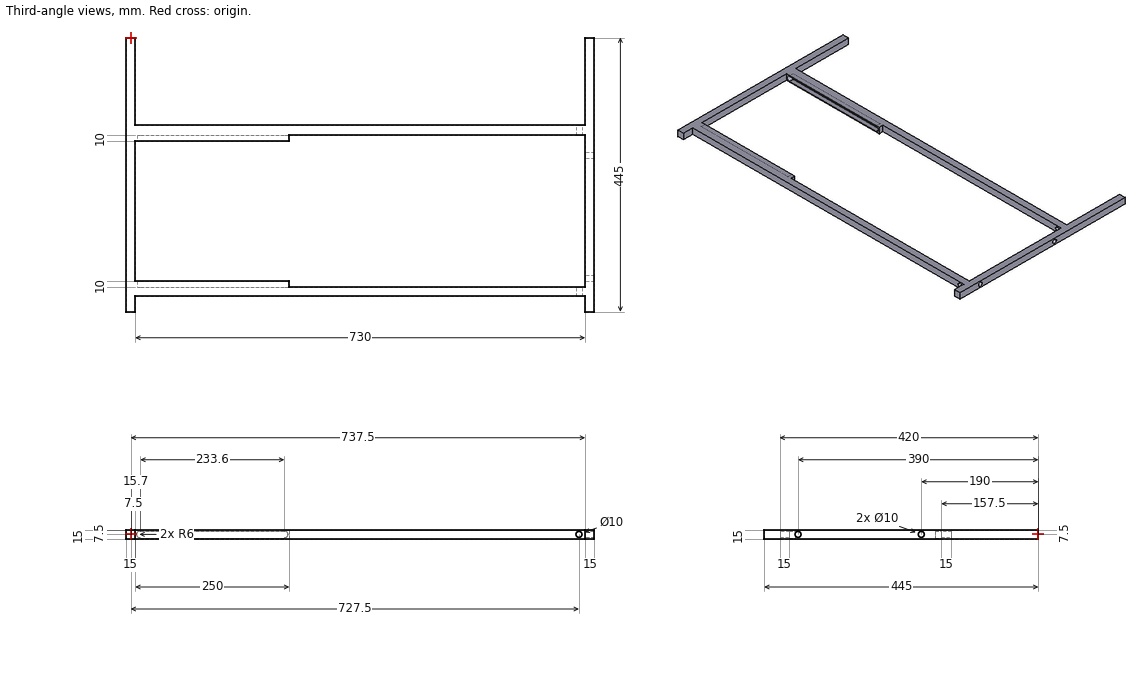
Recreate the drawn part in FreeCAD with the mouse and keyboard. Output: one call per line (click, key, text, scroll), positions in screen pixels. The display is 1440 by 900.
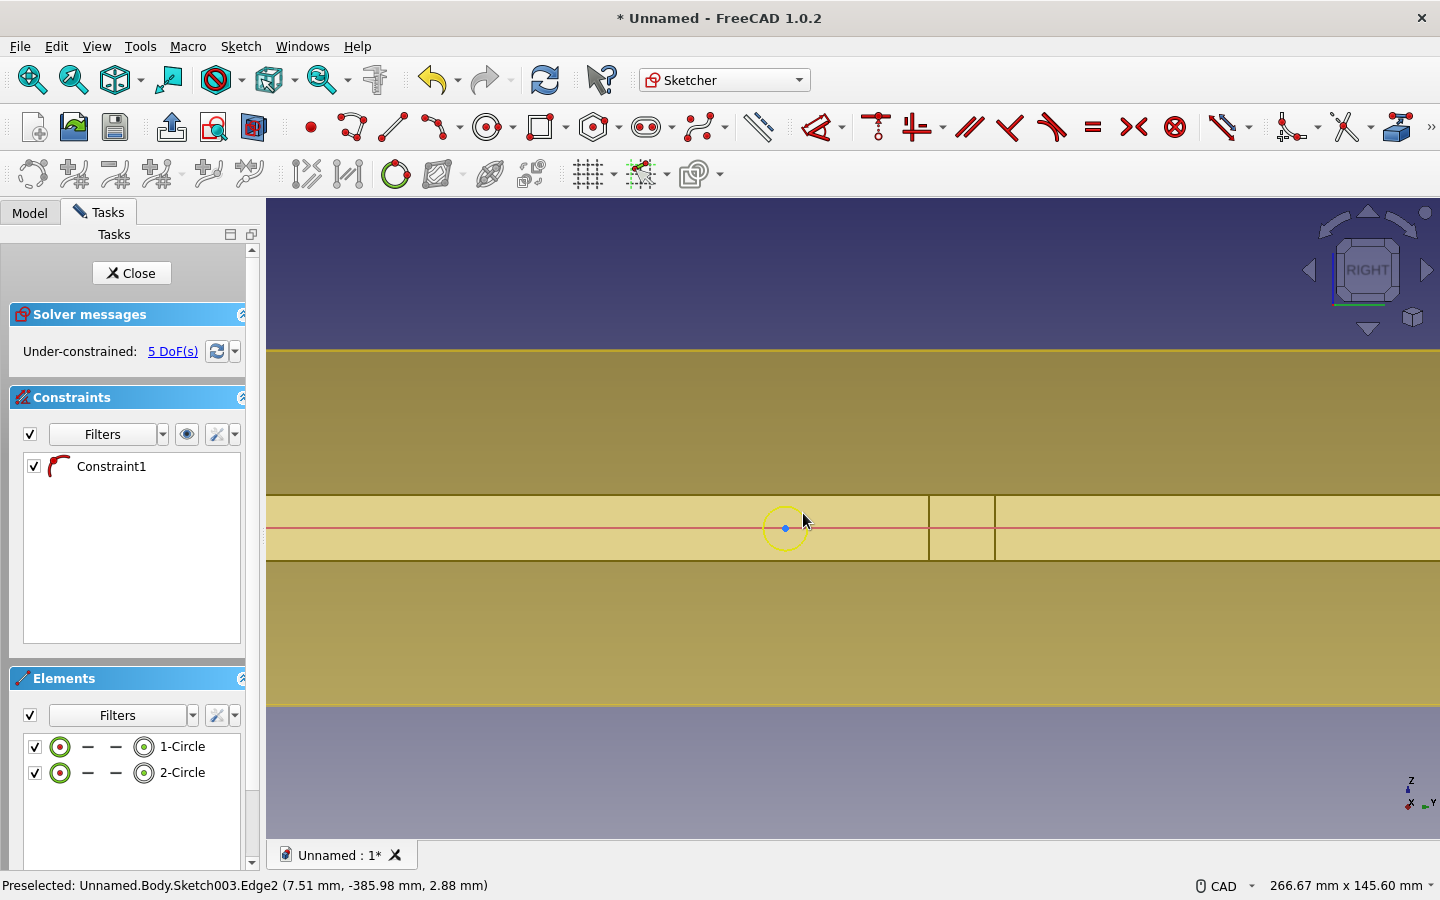
click(801, 513)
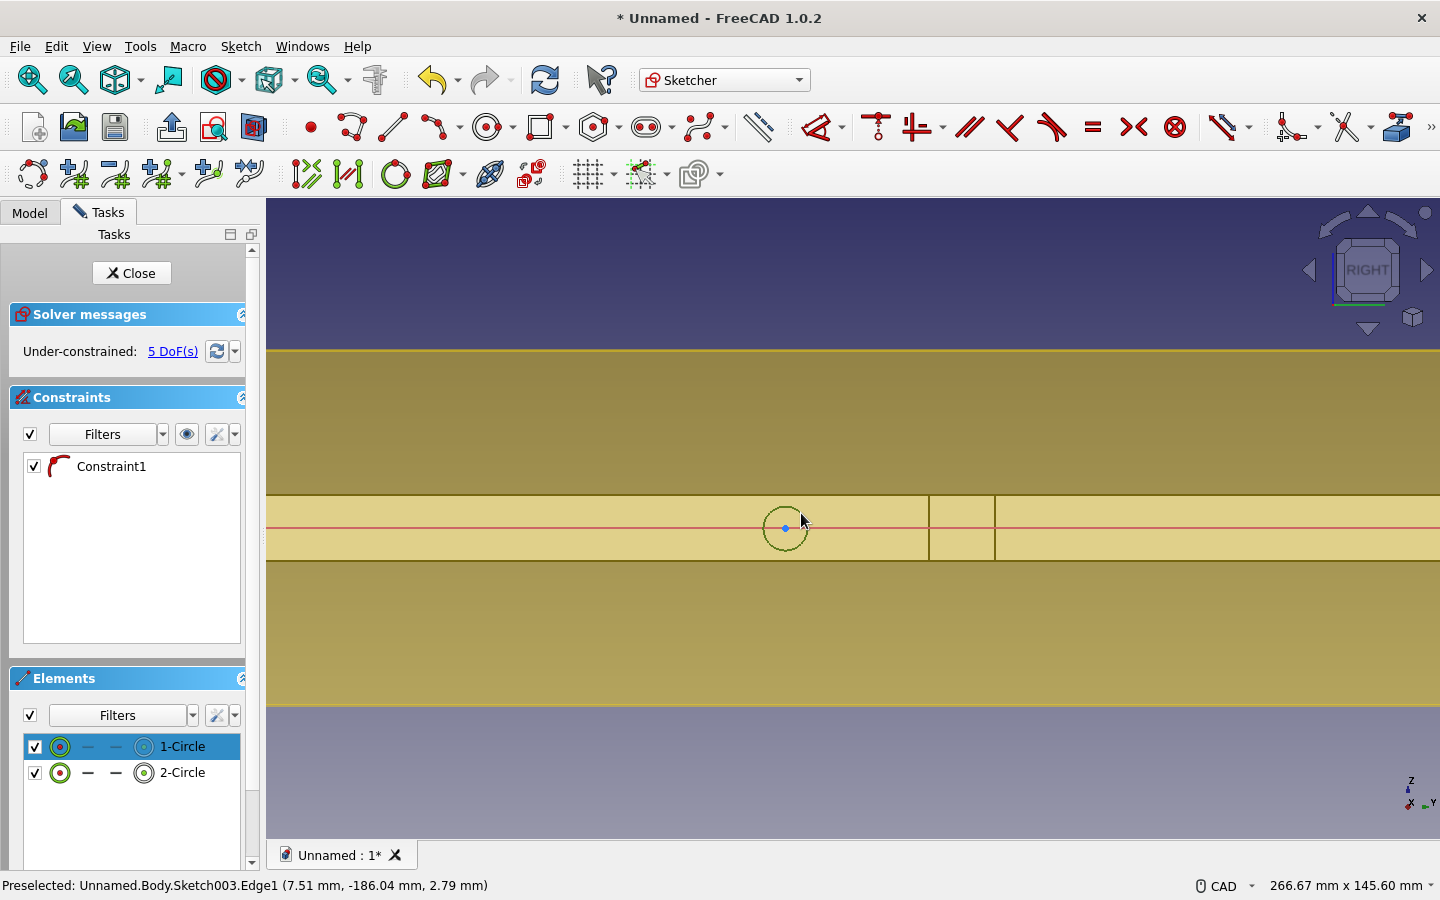
scroll(803, 513, down, 5)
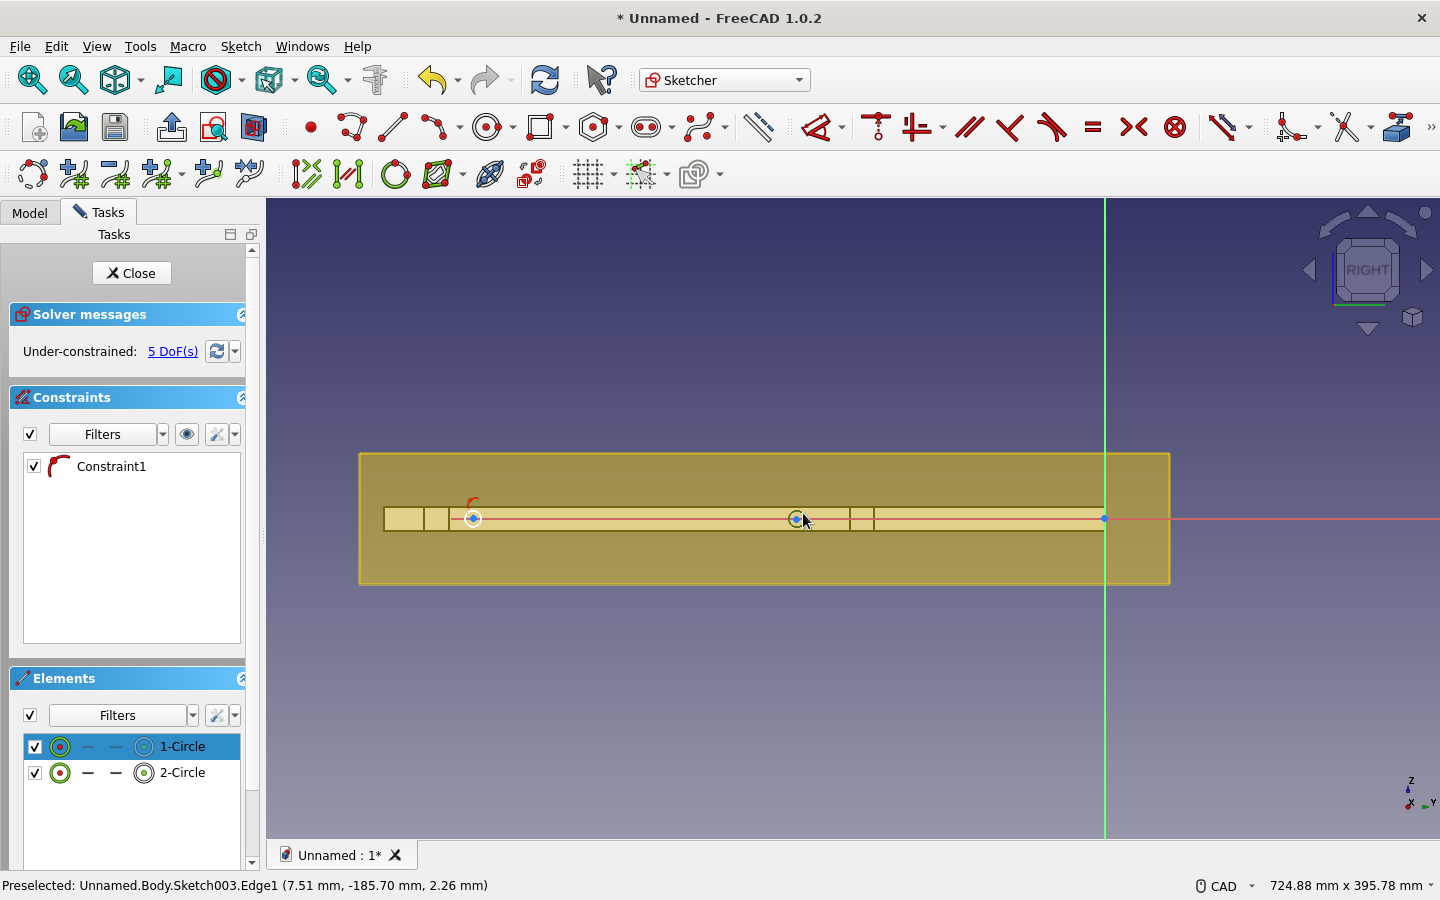
scroll(479, 513, up, 5)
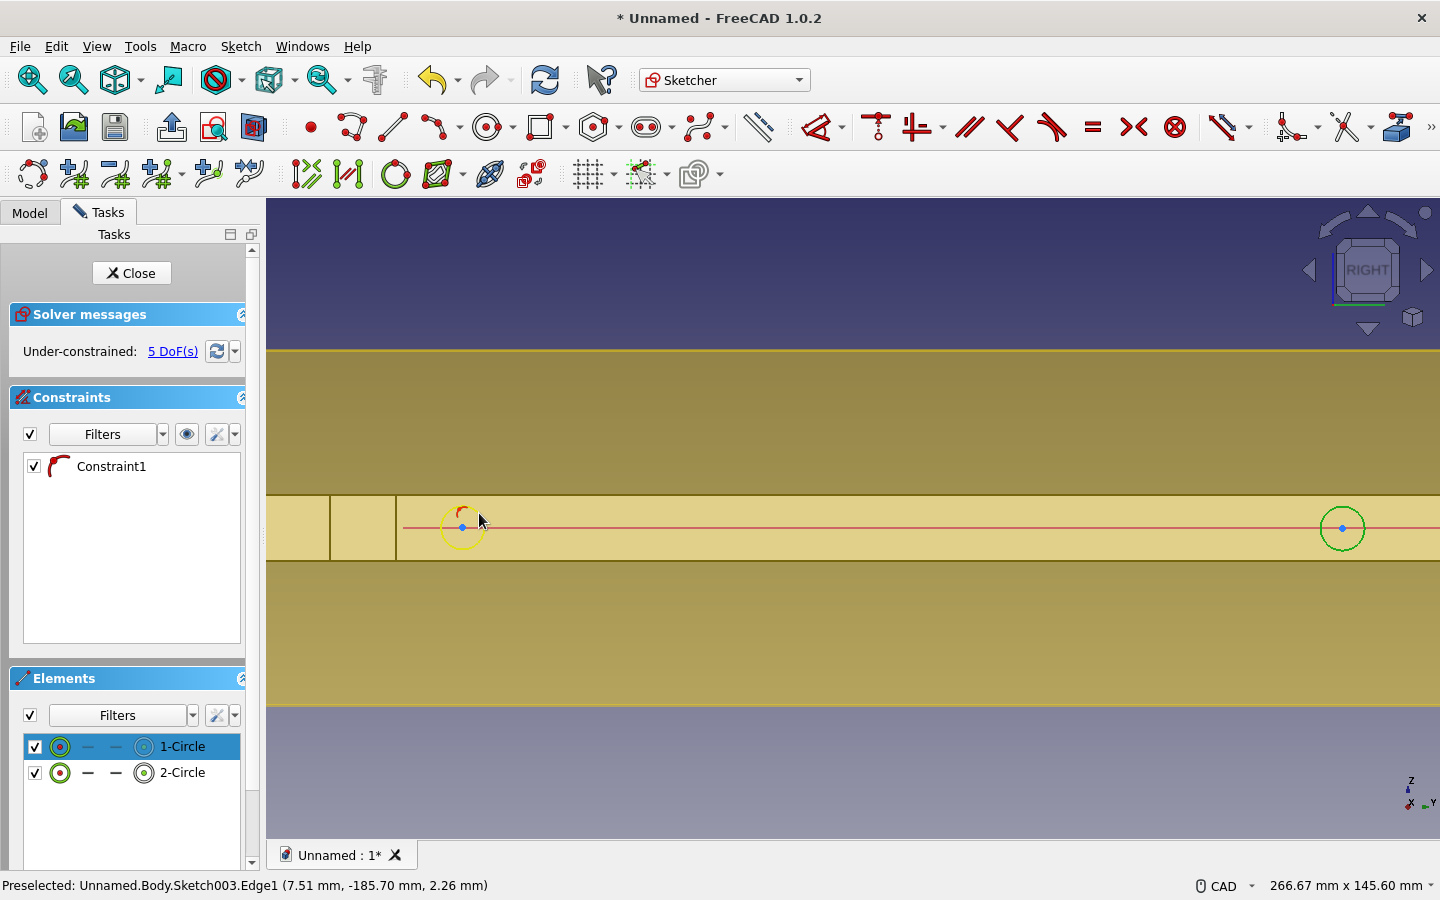
click(478, 513)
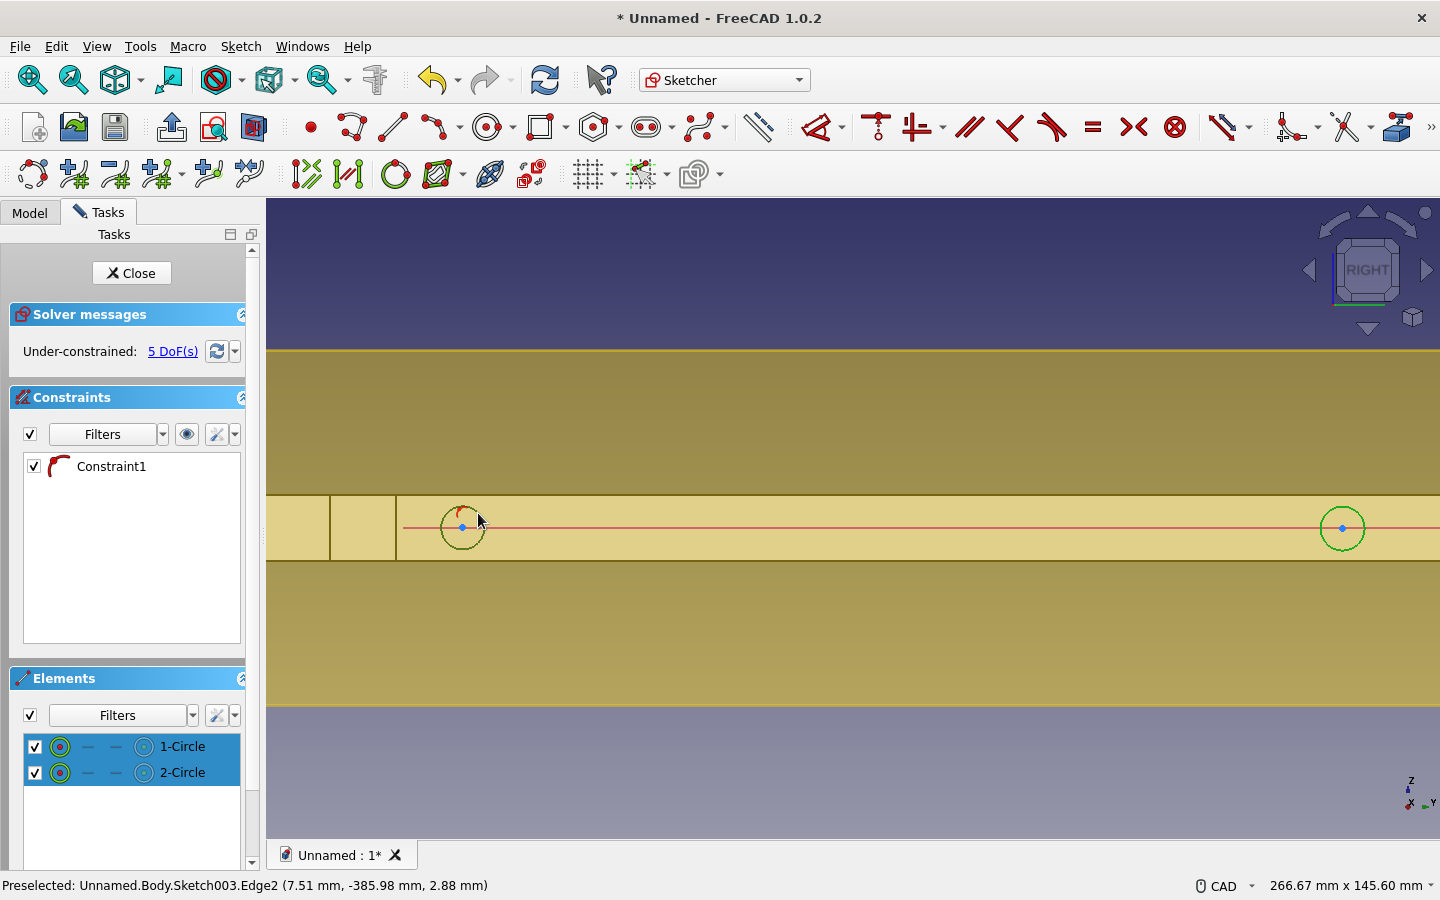
click(1093, 128)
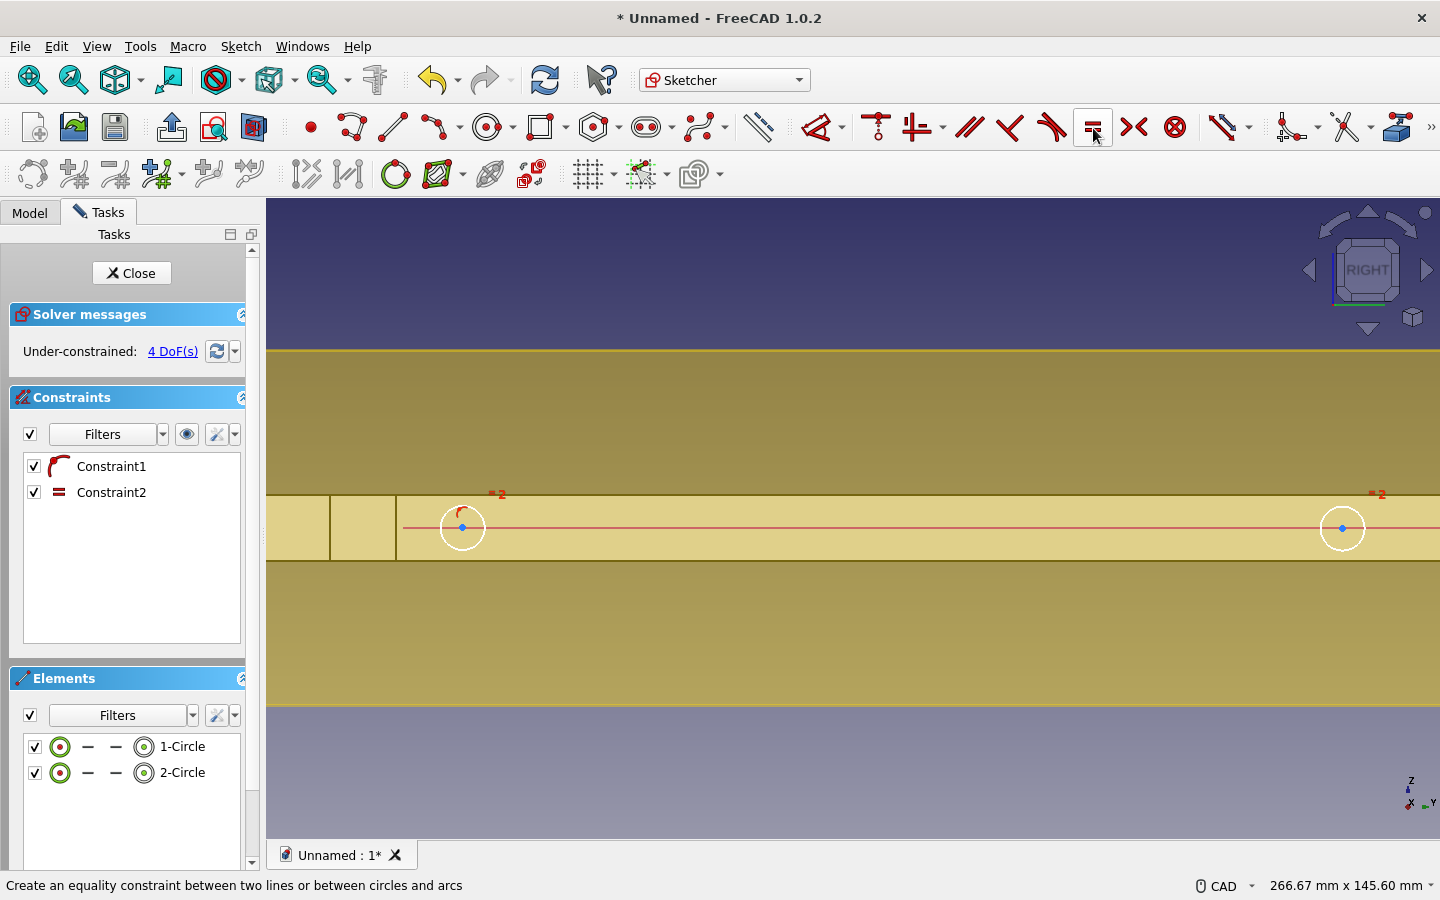
scroll(479, 513, down, 5)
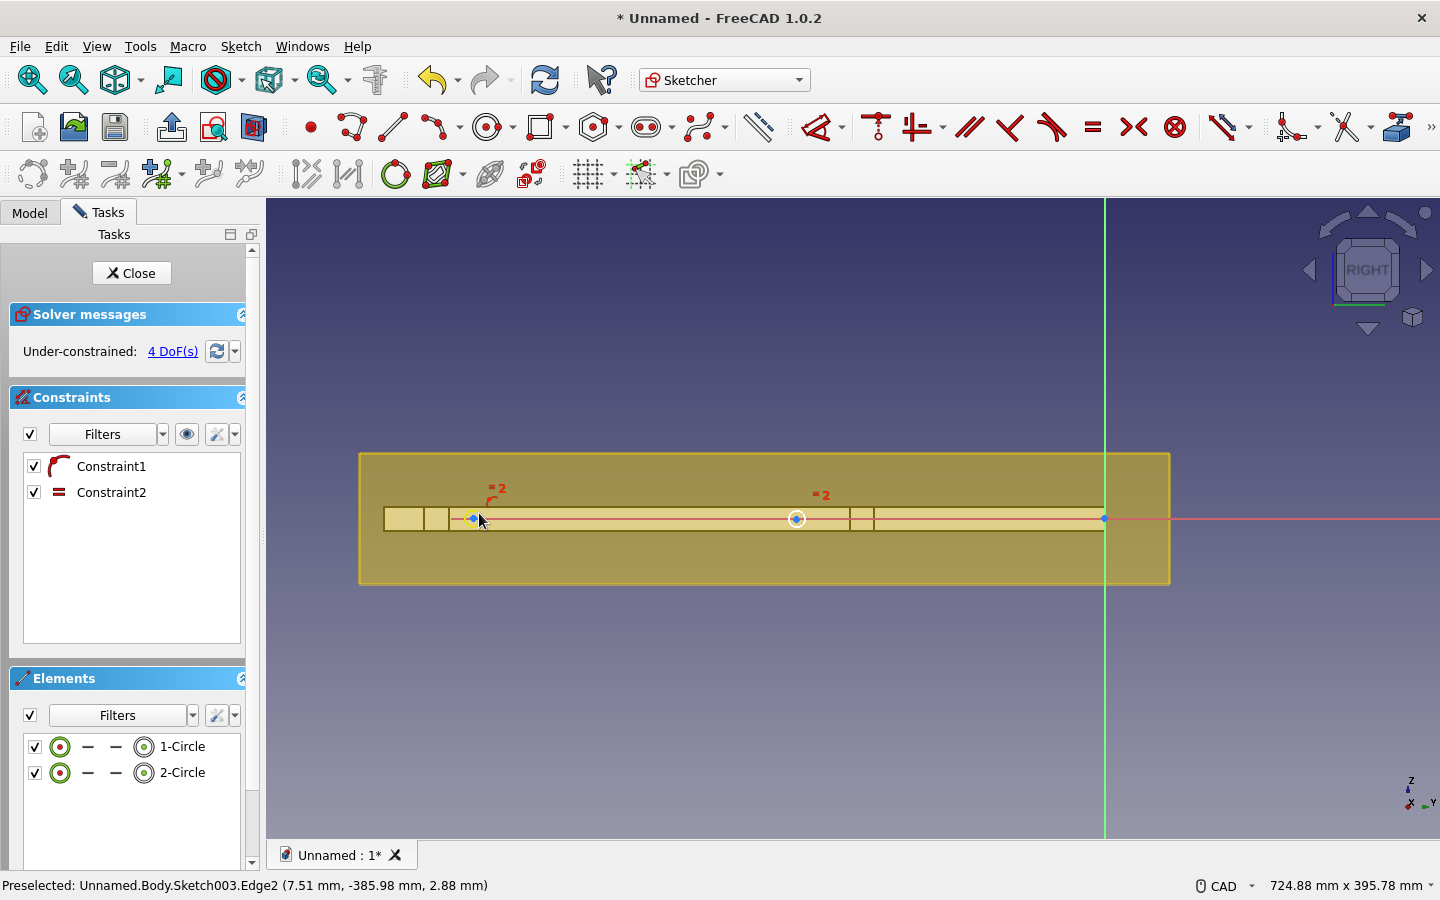
click(797, 519)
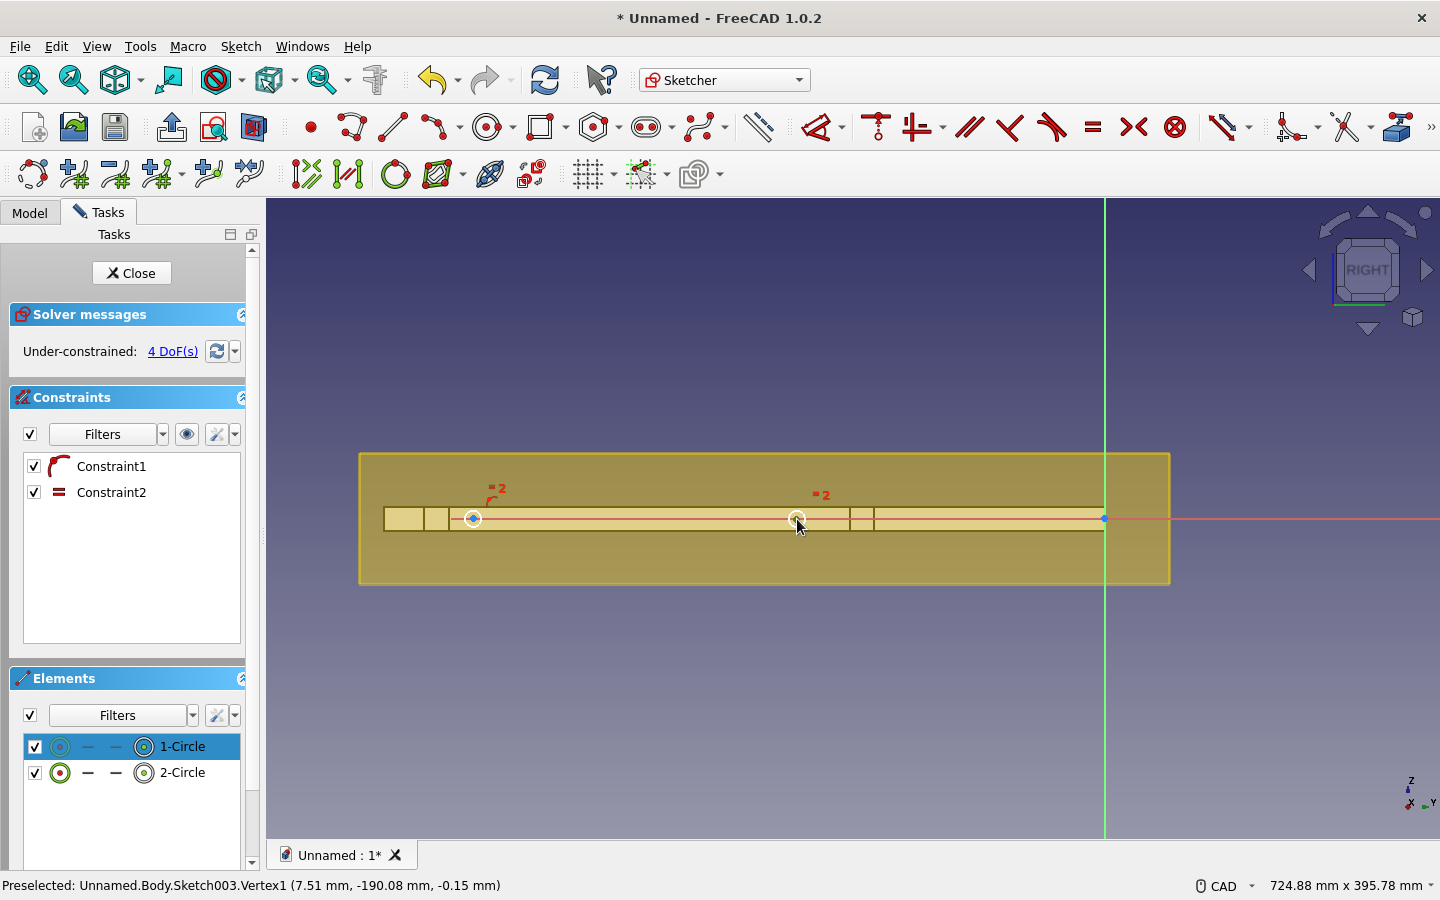
click(574, 519)